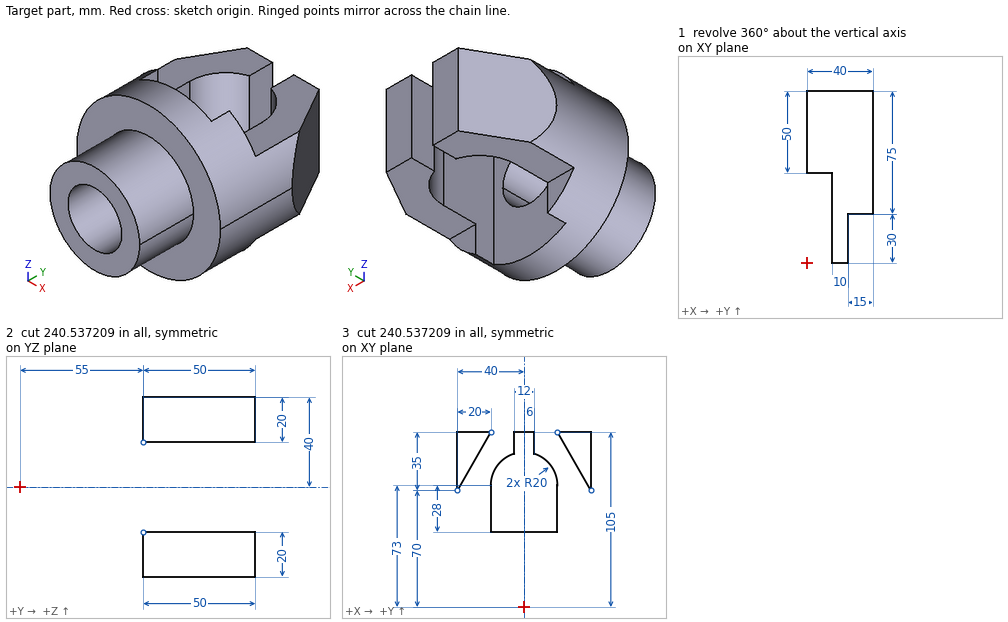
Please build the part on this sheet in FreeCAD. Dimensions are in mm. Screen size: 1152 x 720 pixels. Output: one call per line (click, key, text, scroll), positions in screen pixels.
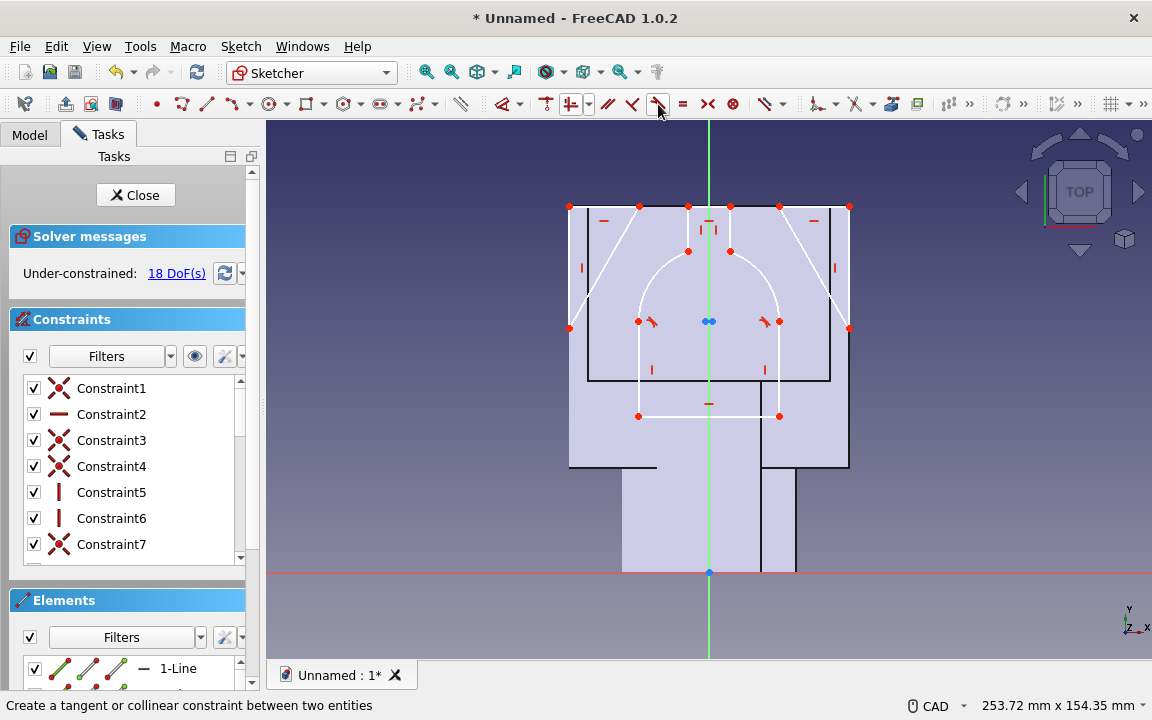
click(665, 265)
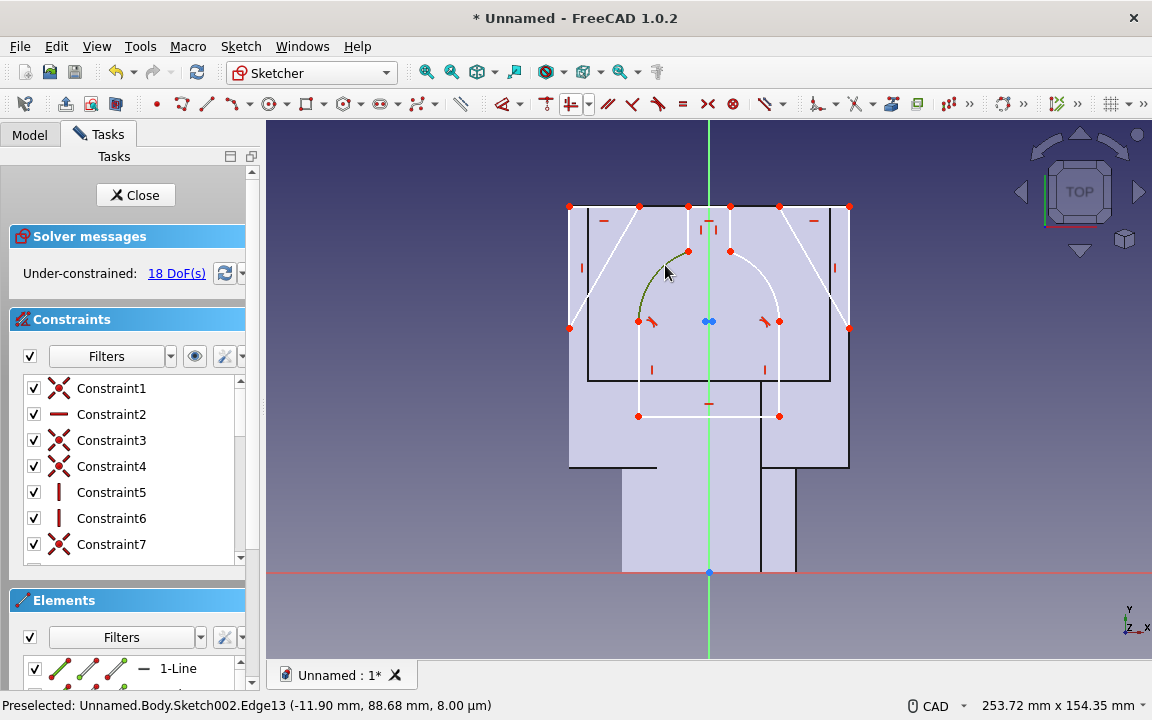
click(774, 295)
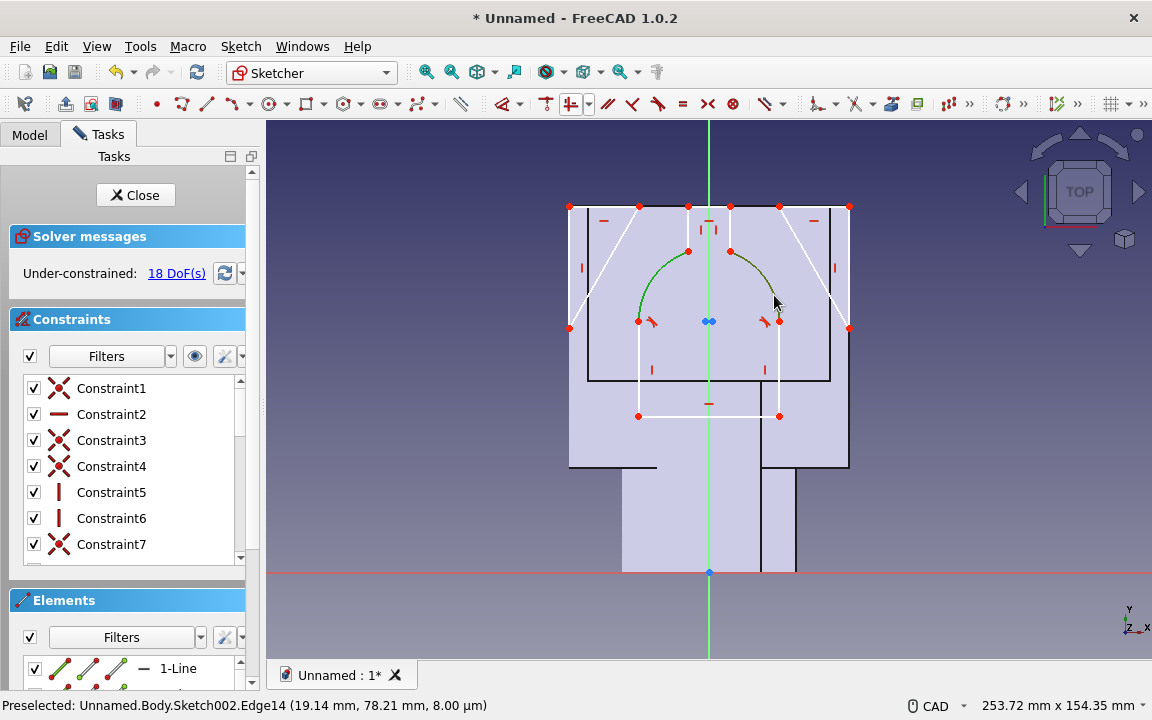
click(546, 104)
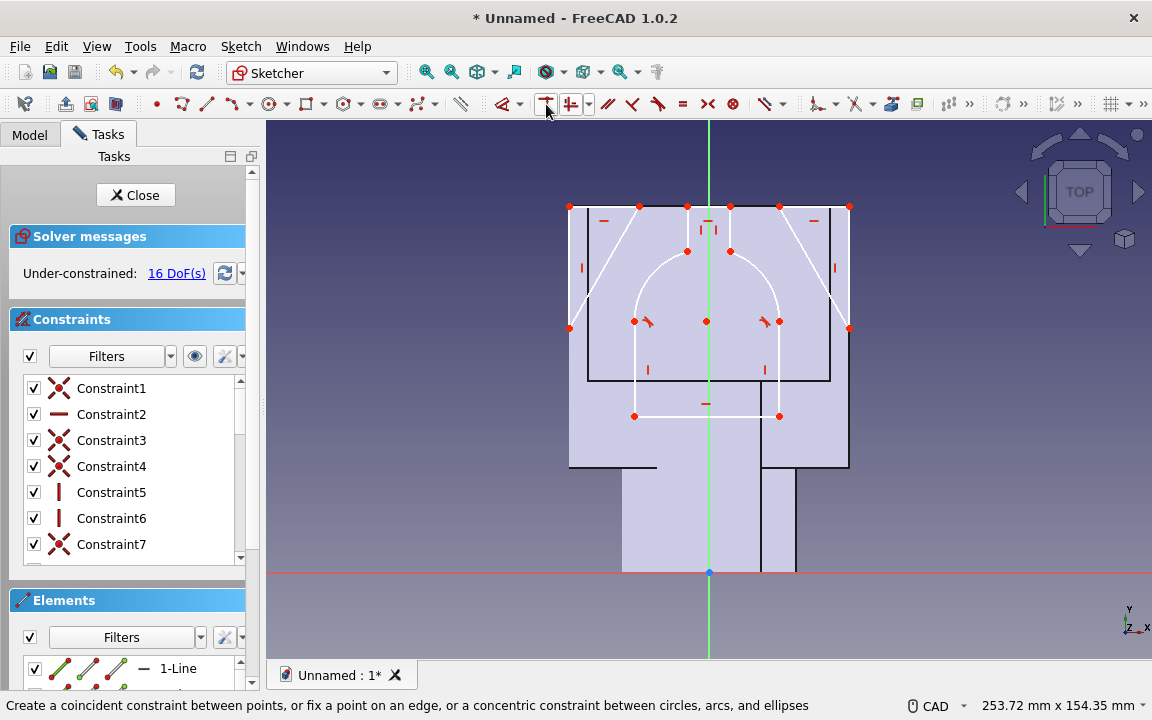
click(663, 264)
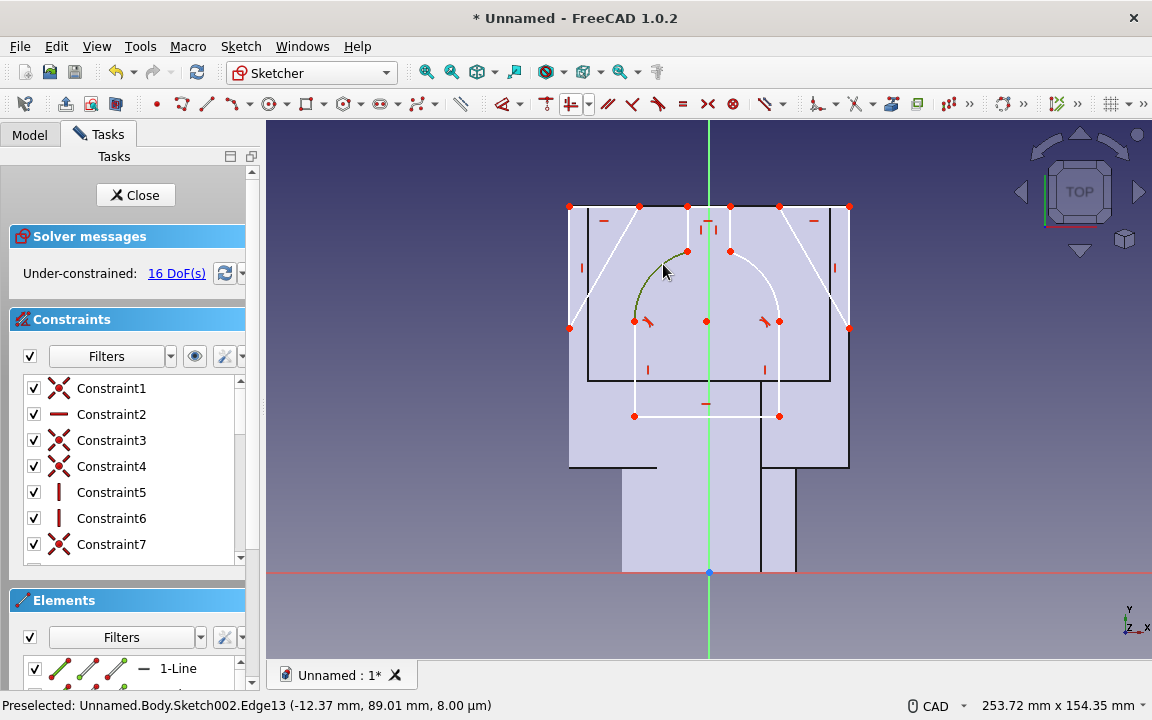
click(774, 295)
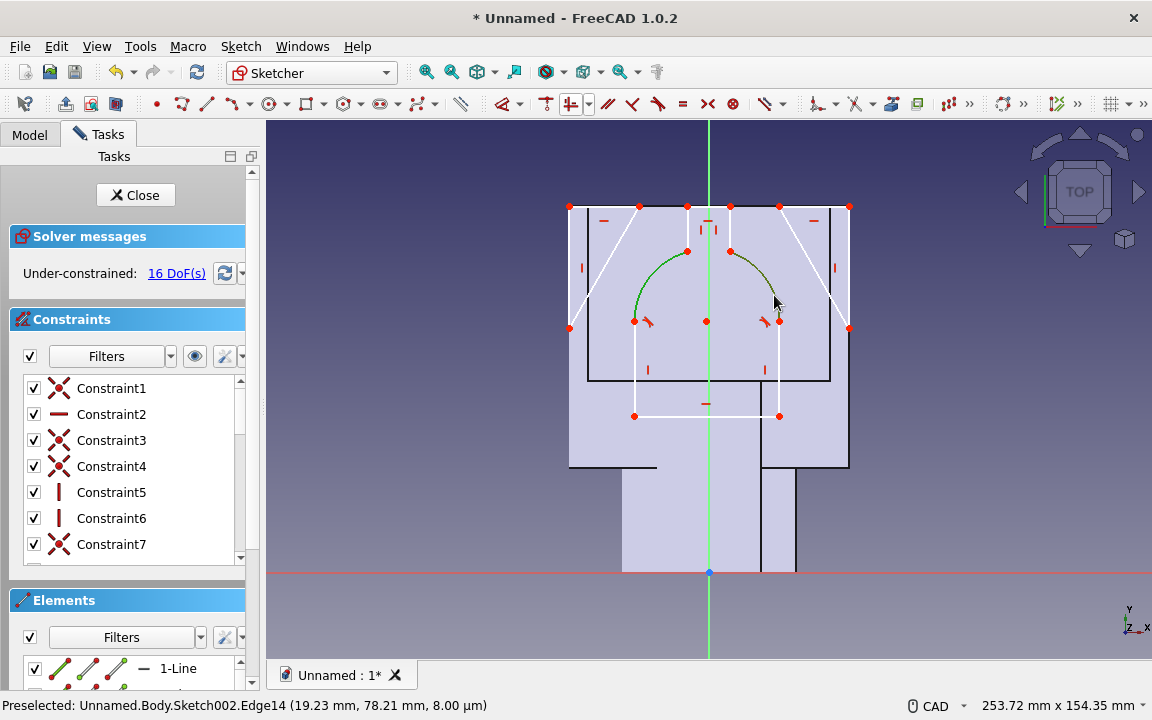
click(683, 104)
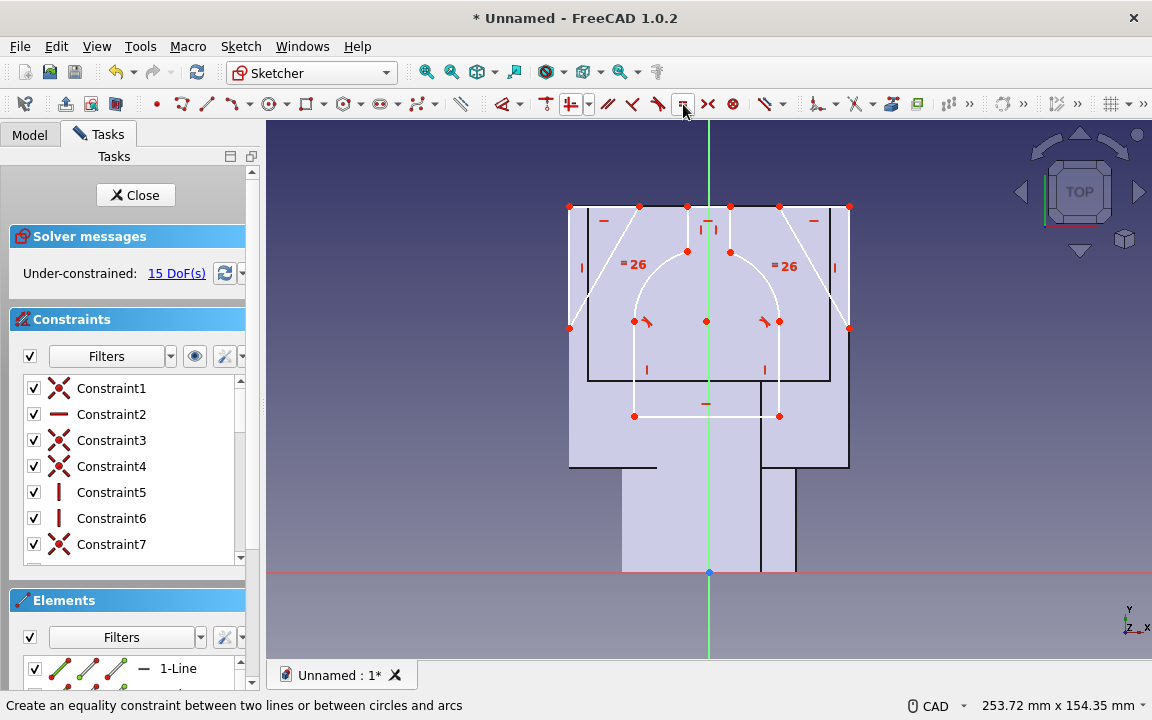
click(707, 322)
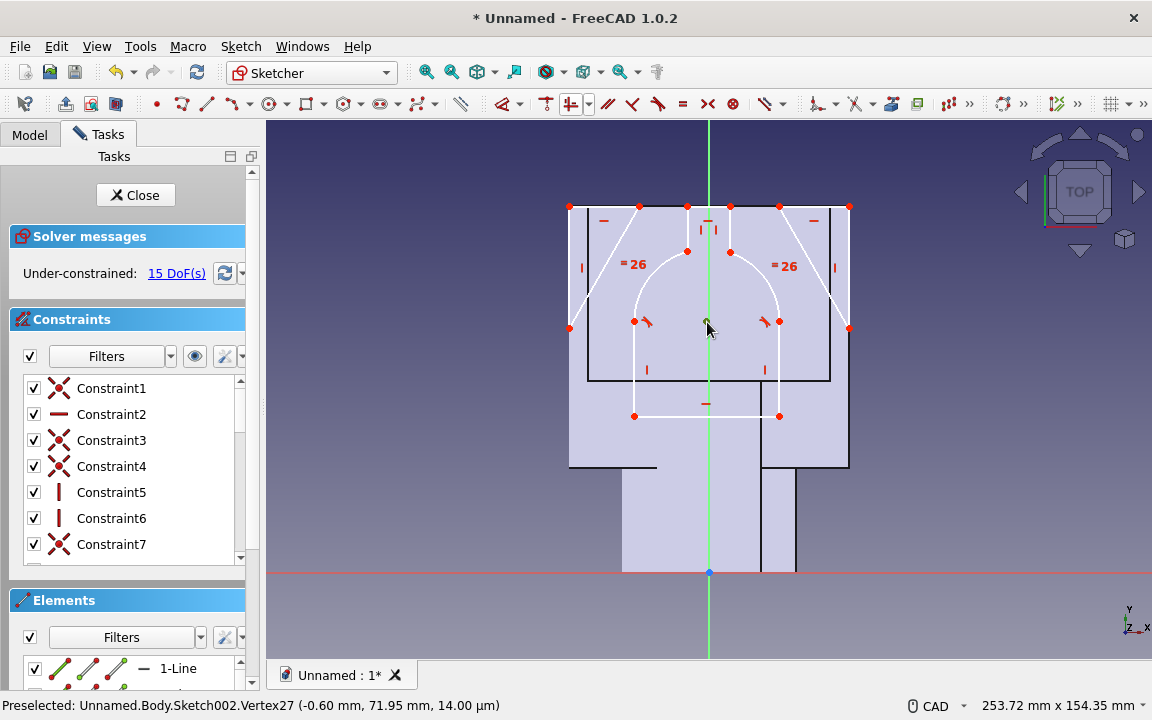
click(709, 528)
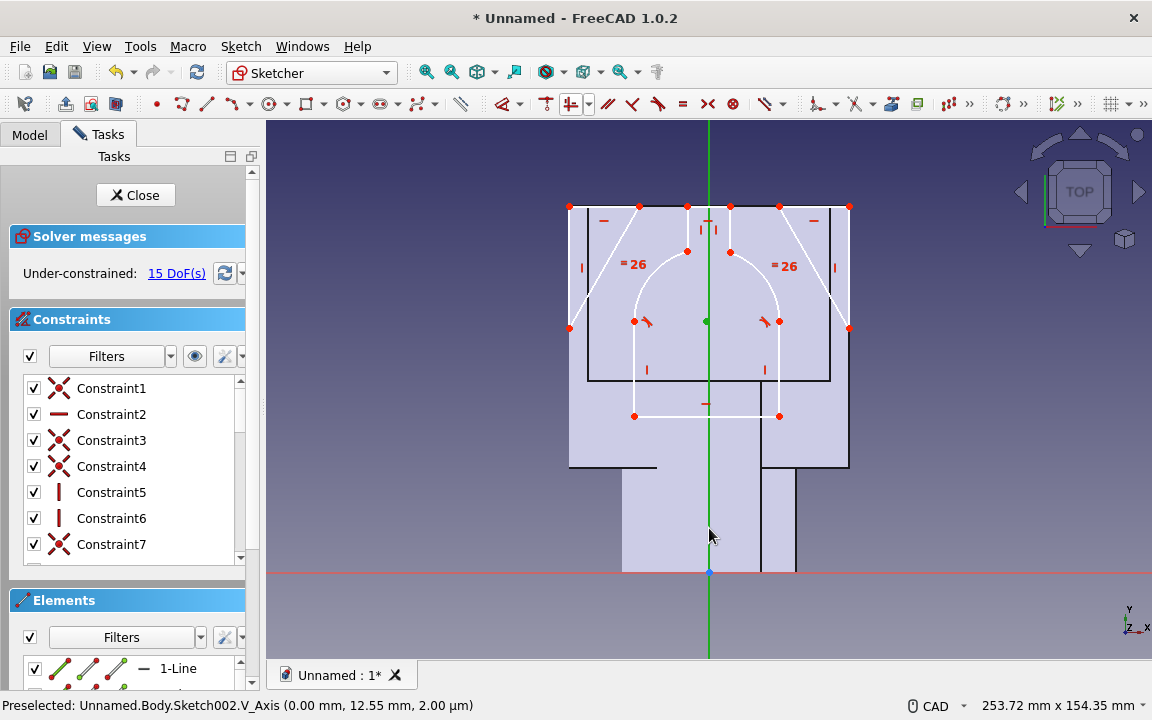
click(546, 104)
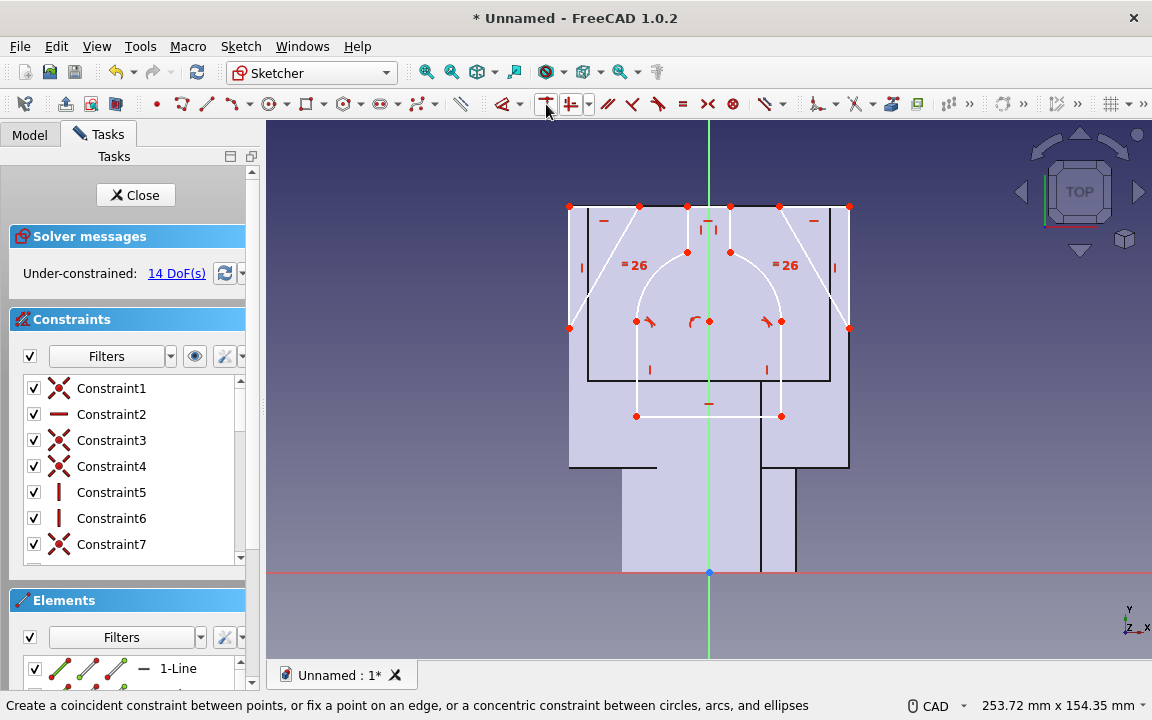
click(569, 329)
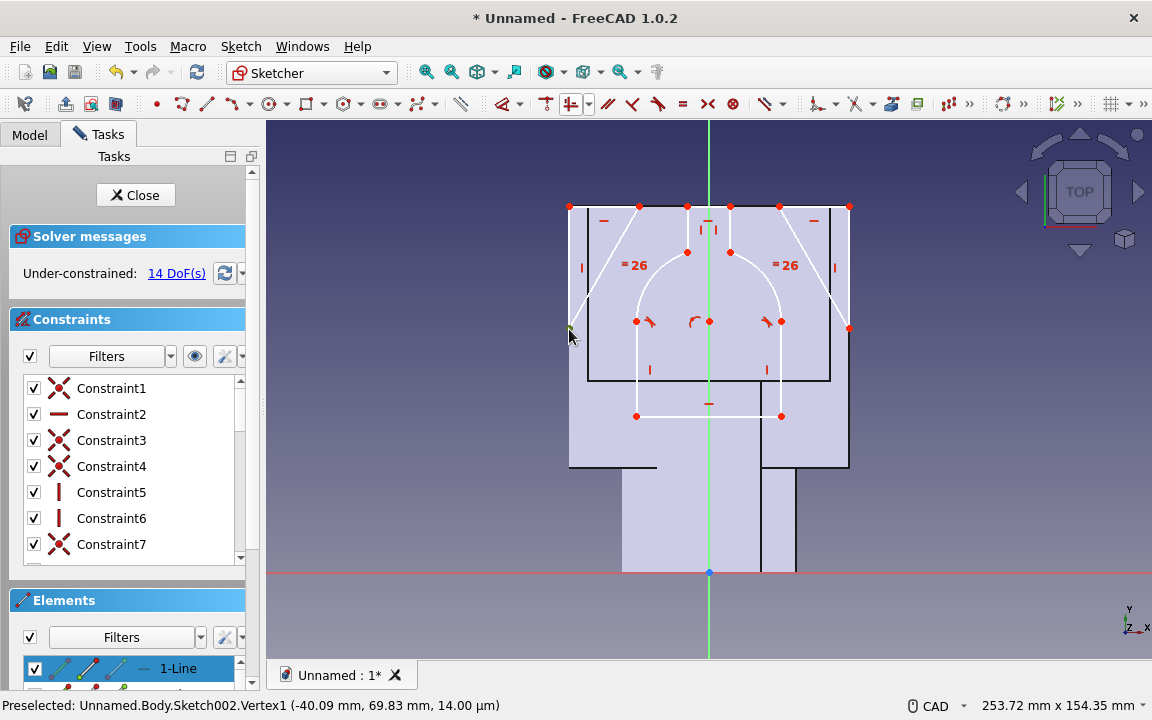
click(849, 329)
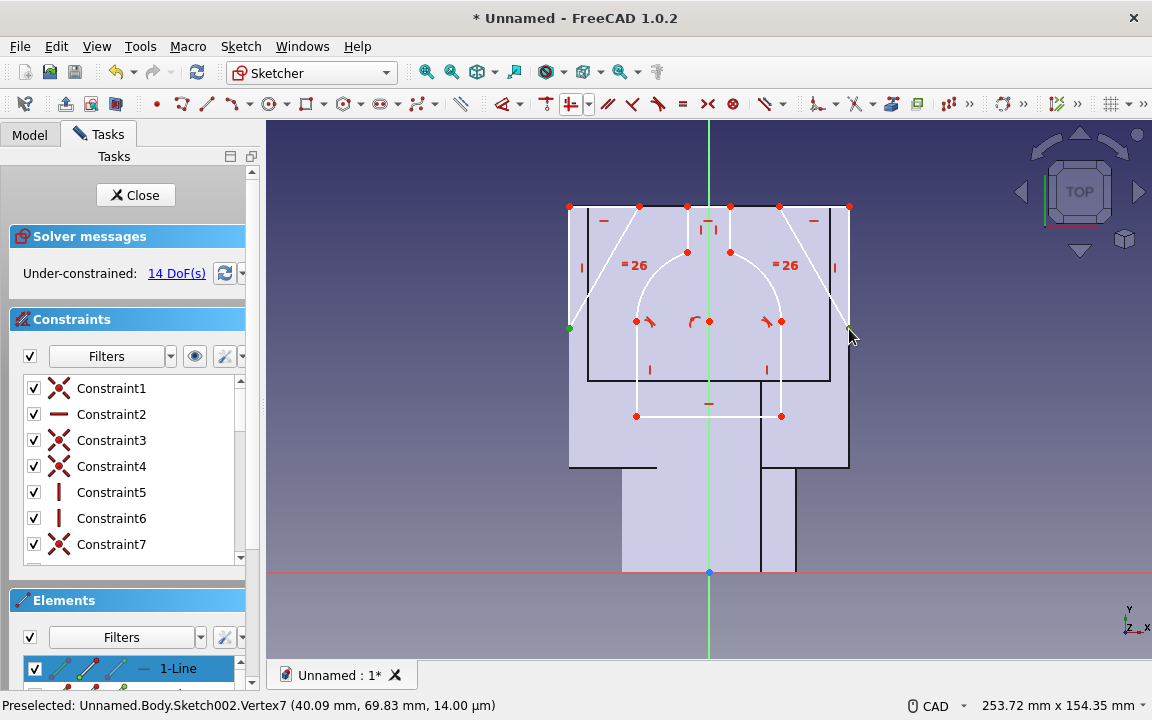
click(709, 528)